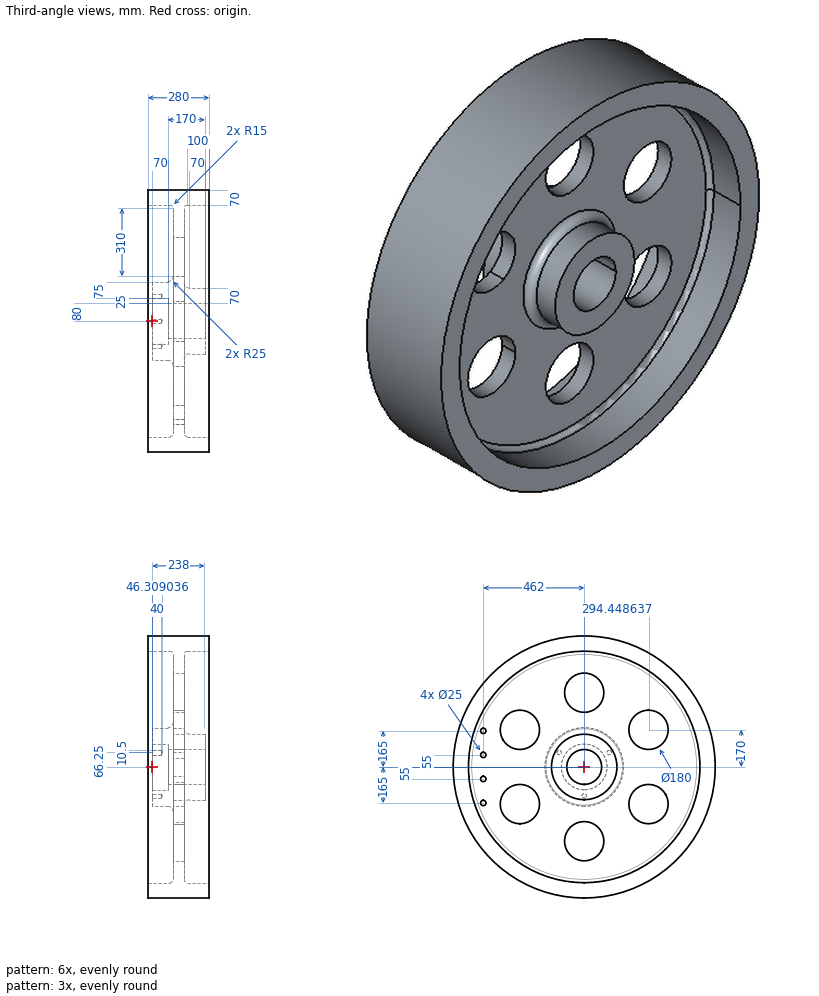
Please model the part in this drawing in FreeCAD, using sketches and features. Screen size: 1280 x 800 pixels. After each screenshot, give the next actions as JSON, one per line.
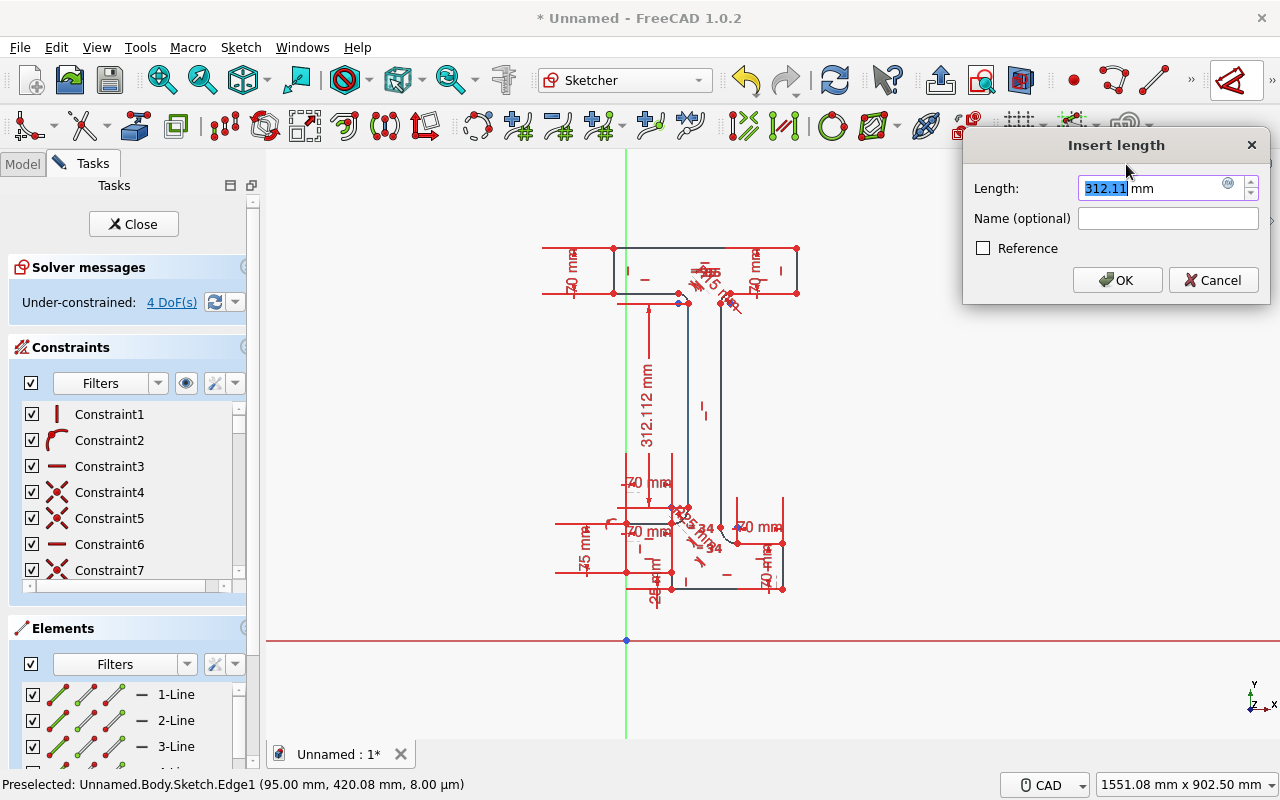
{"action": "type", "text": "310"}
{"action": "key", "text": "Return"}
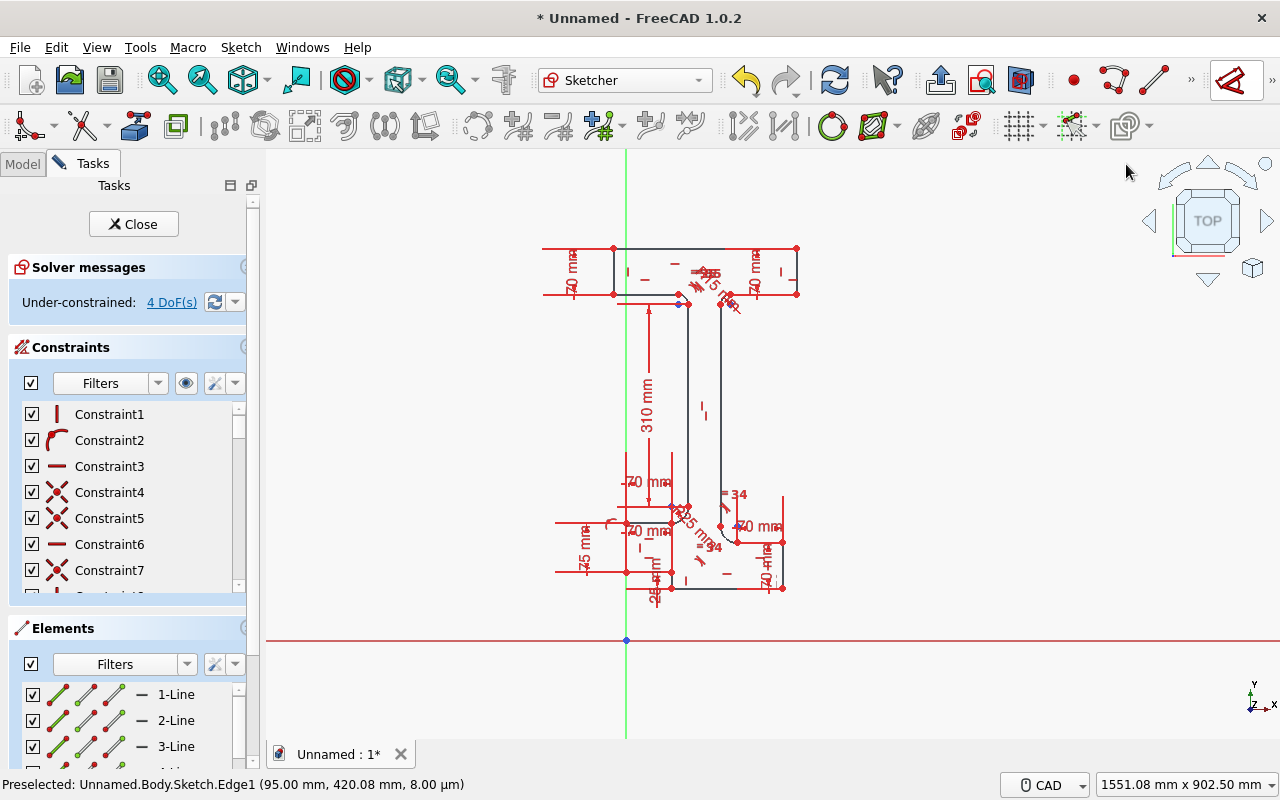
{"action": "left_click", "coordinate": [705, 589]}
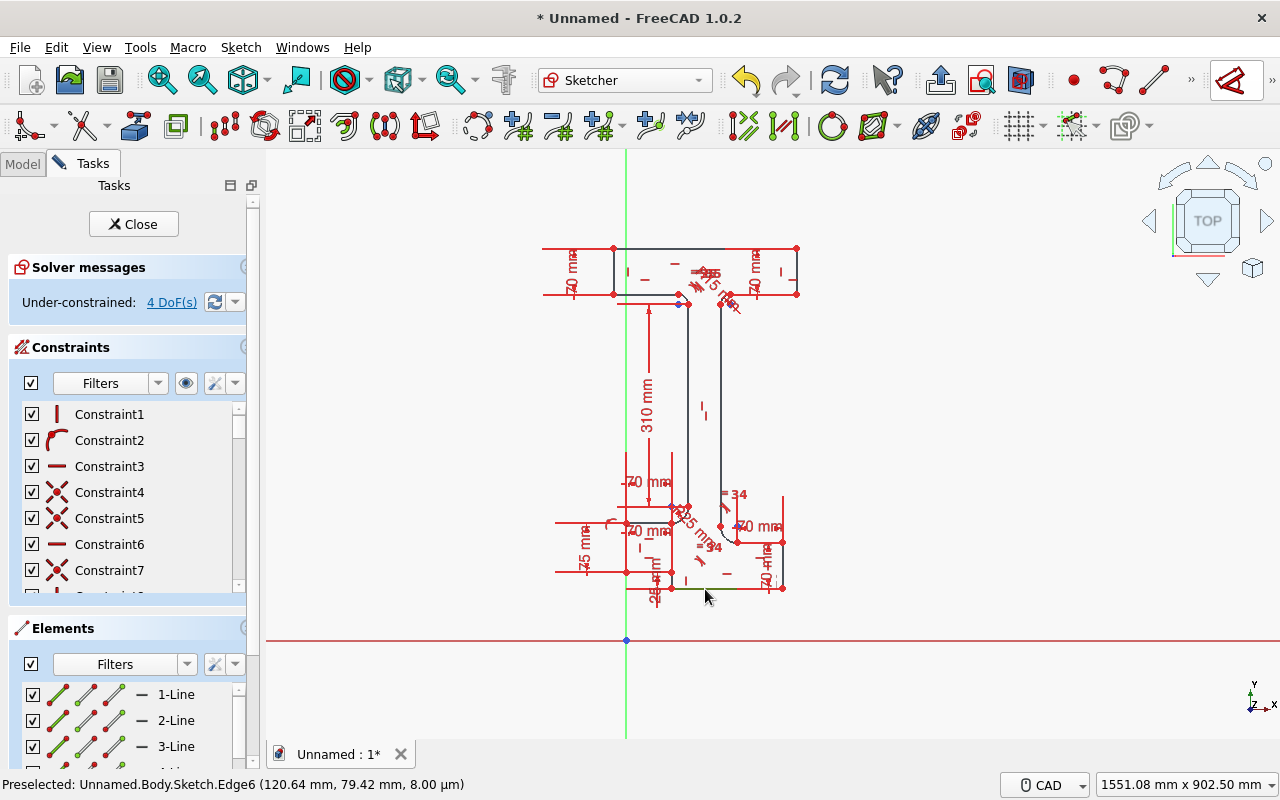
{"action": "left_click", "coordinate": [1258, 80]}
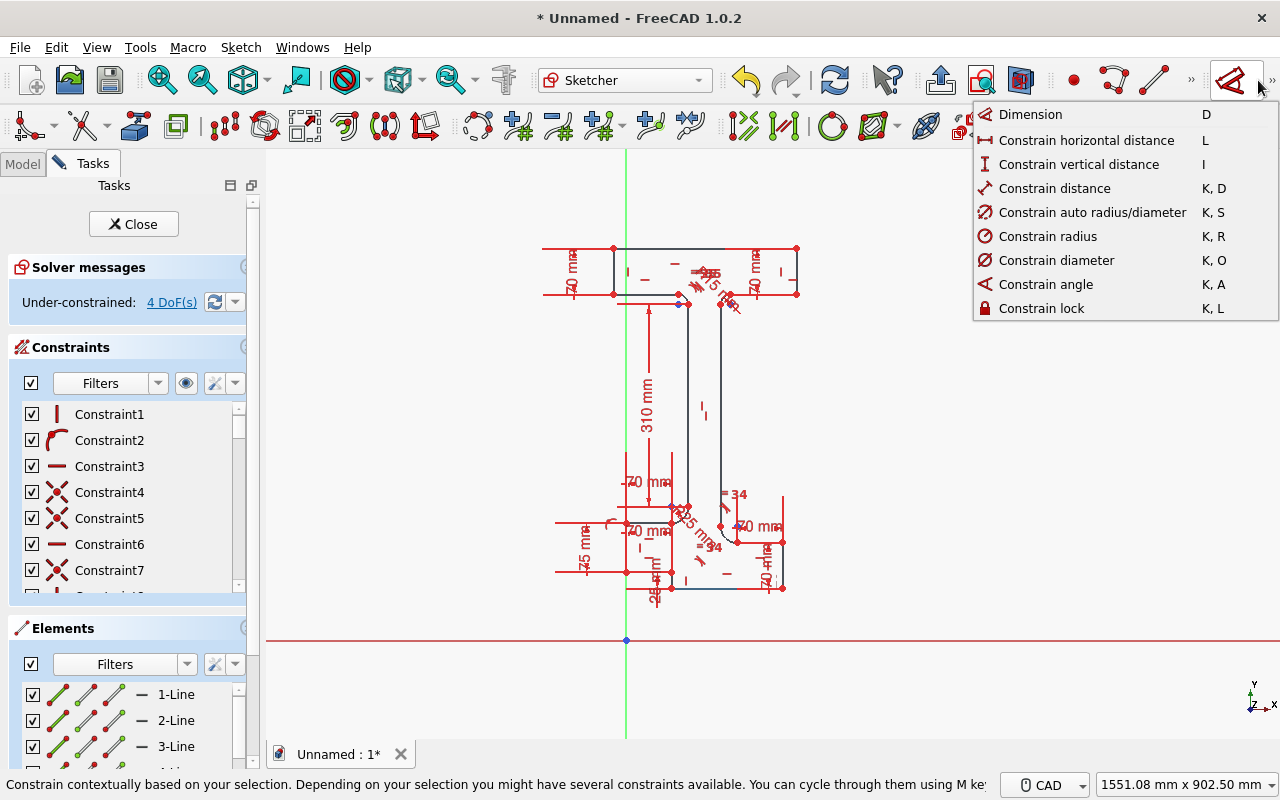
{"action": "left_click", "coordinate": [1126, 140]}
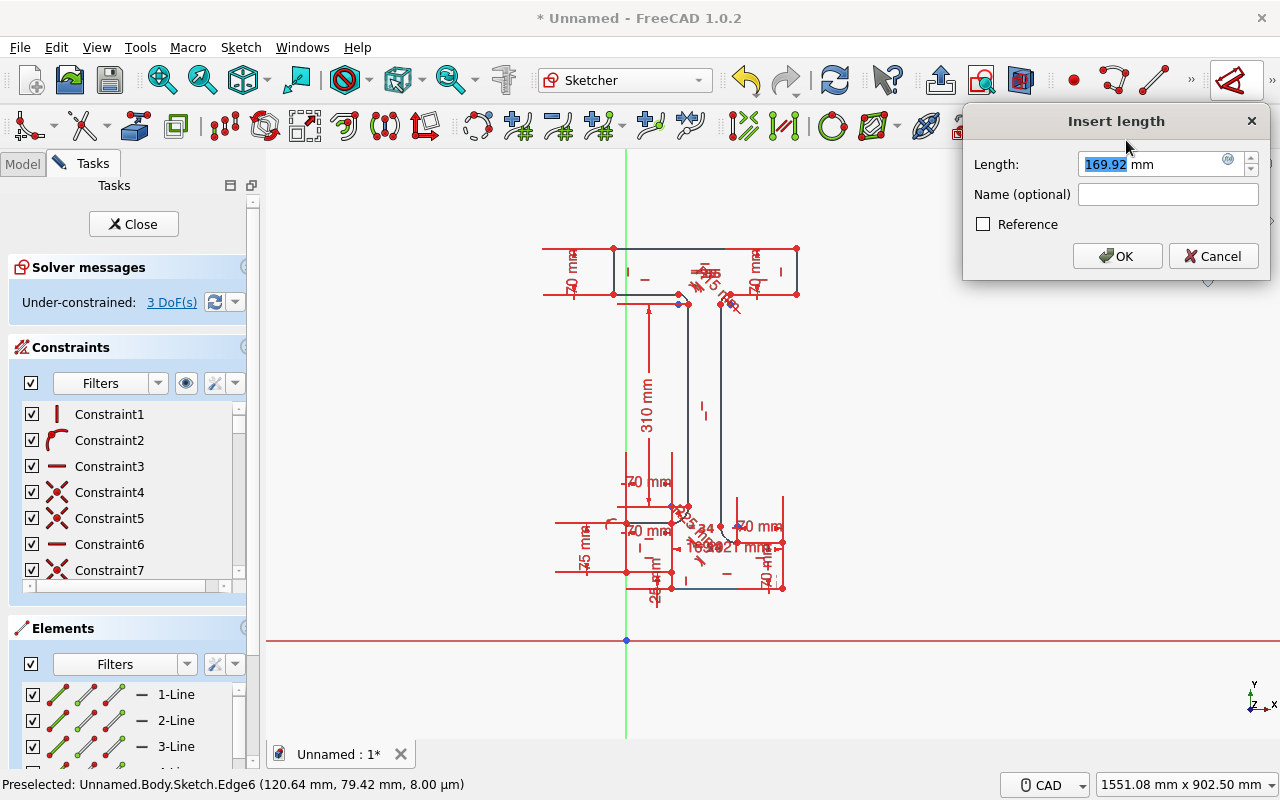
{"action": "type", "text": "170"}
{"action": "key", "text": "Return"}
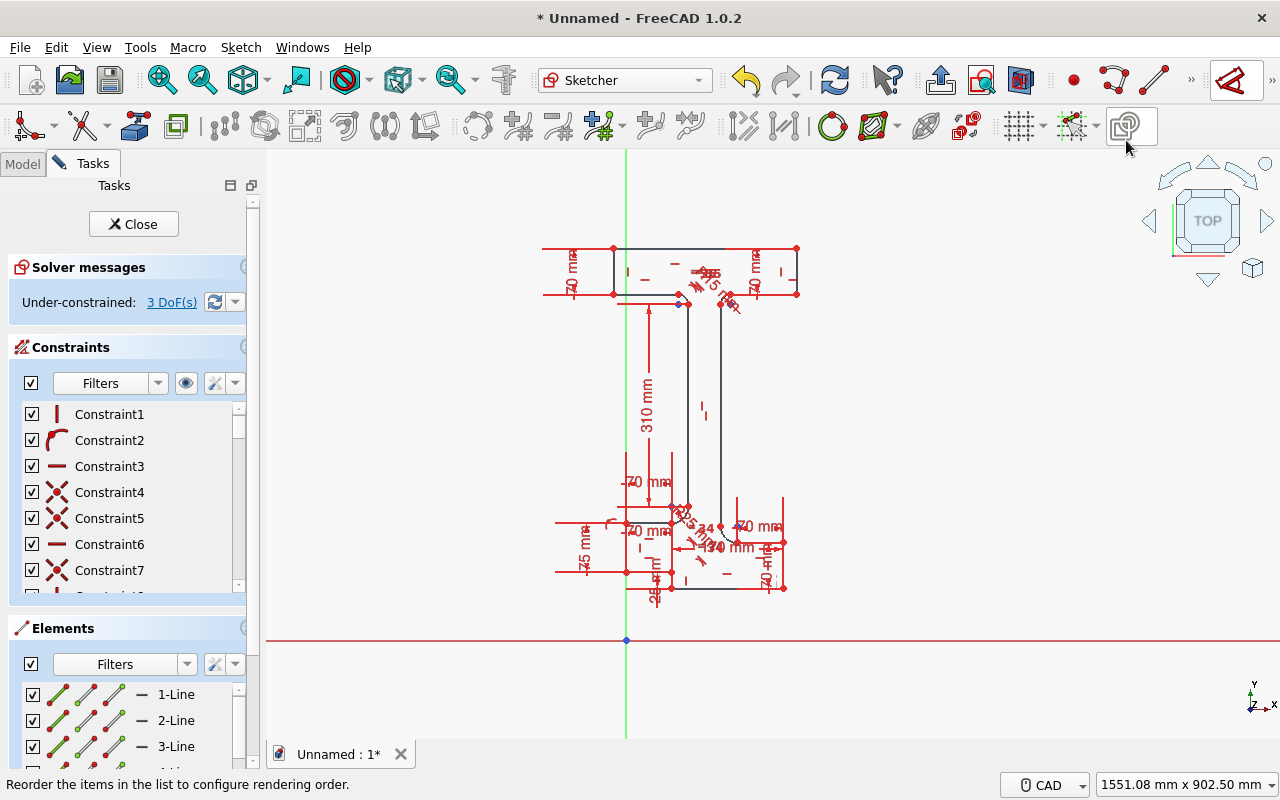
{"action": "left_click", "coordinate": [750, 295]}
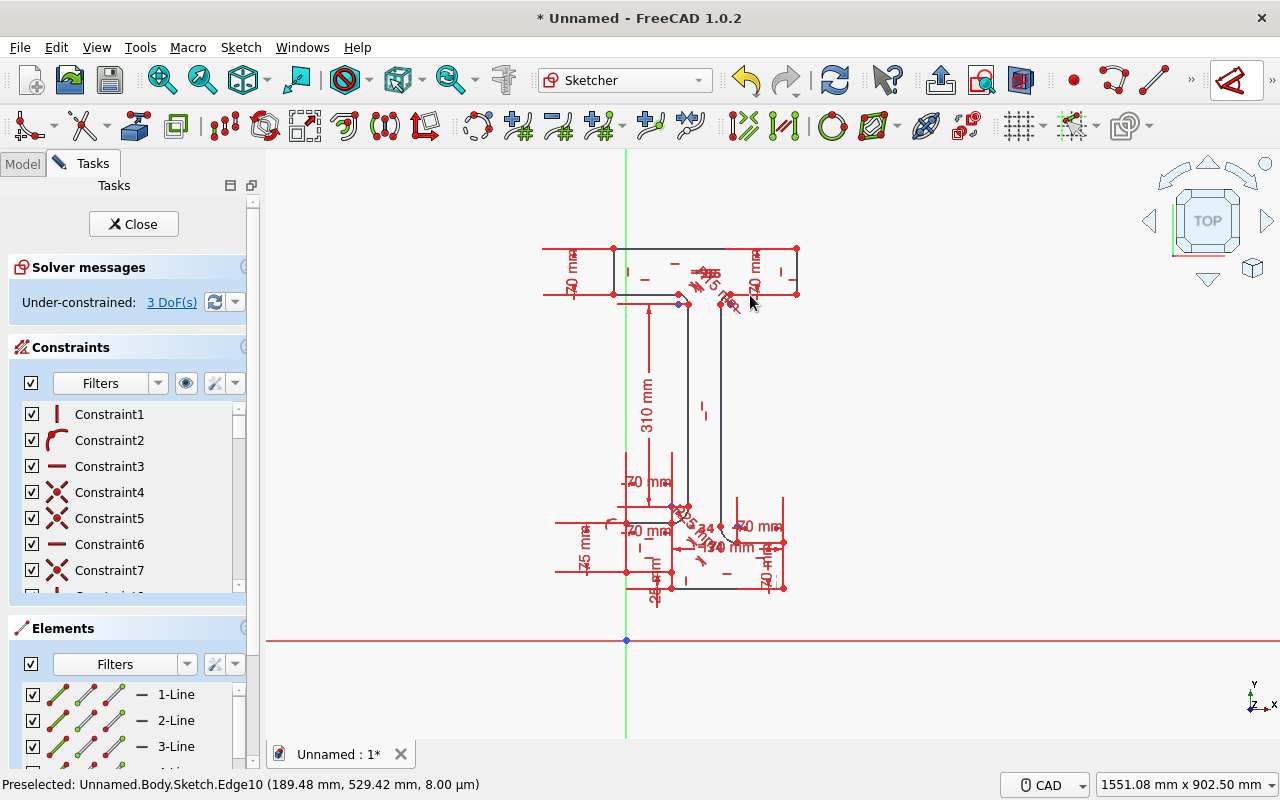
{"action": "left_click", "coordinate": [1258, 80]}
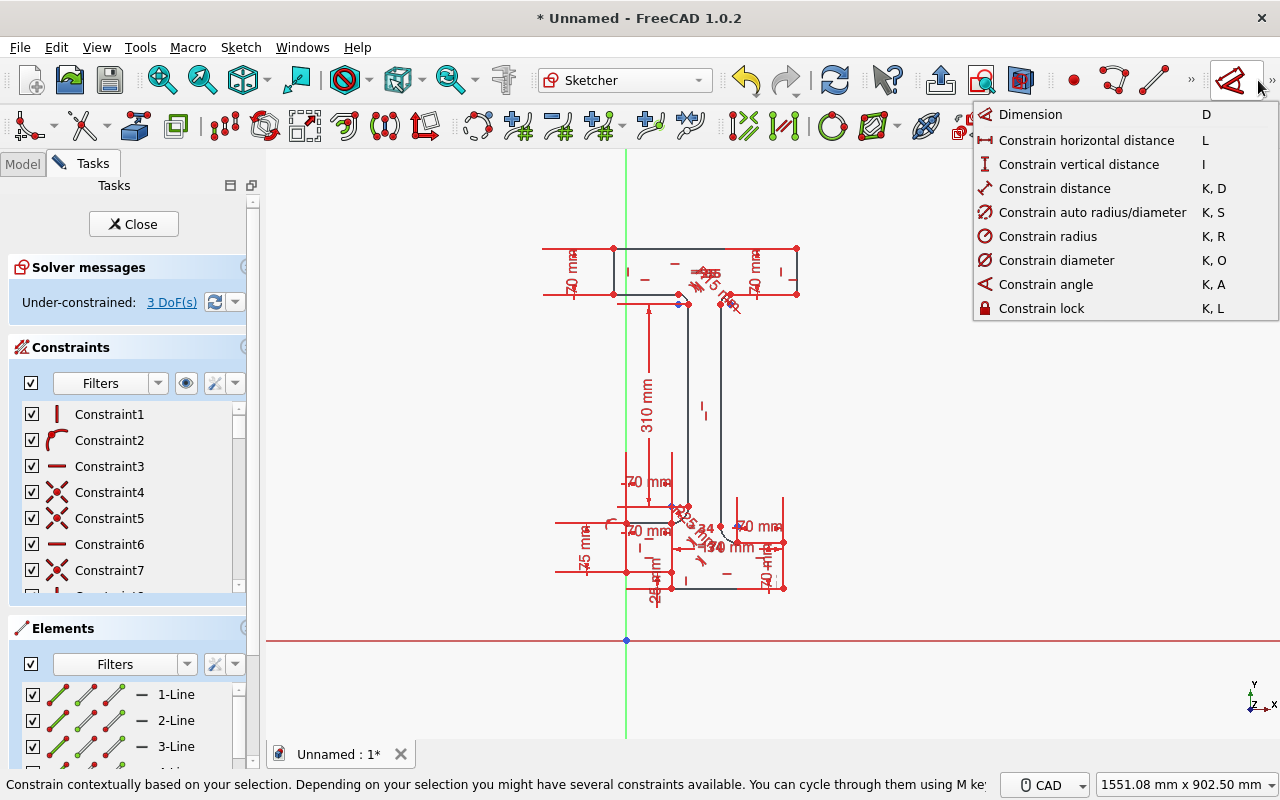
{"action": "left_click", "coordinate": [1126, 140]}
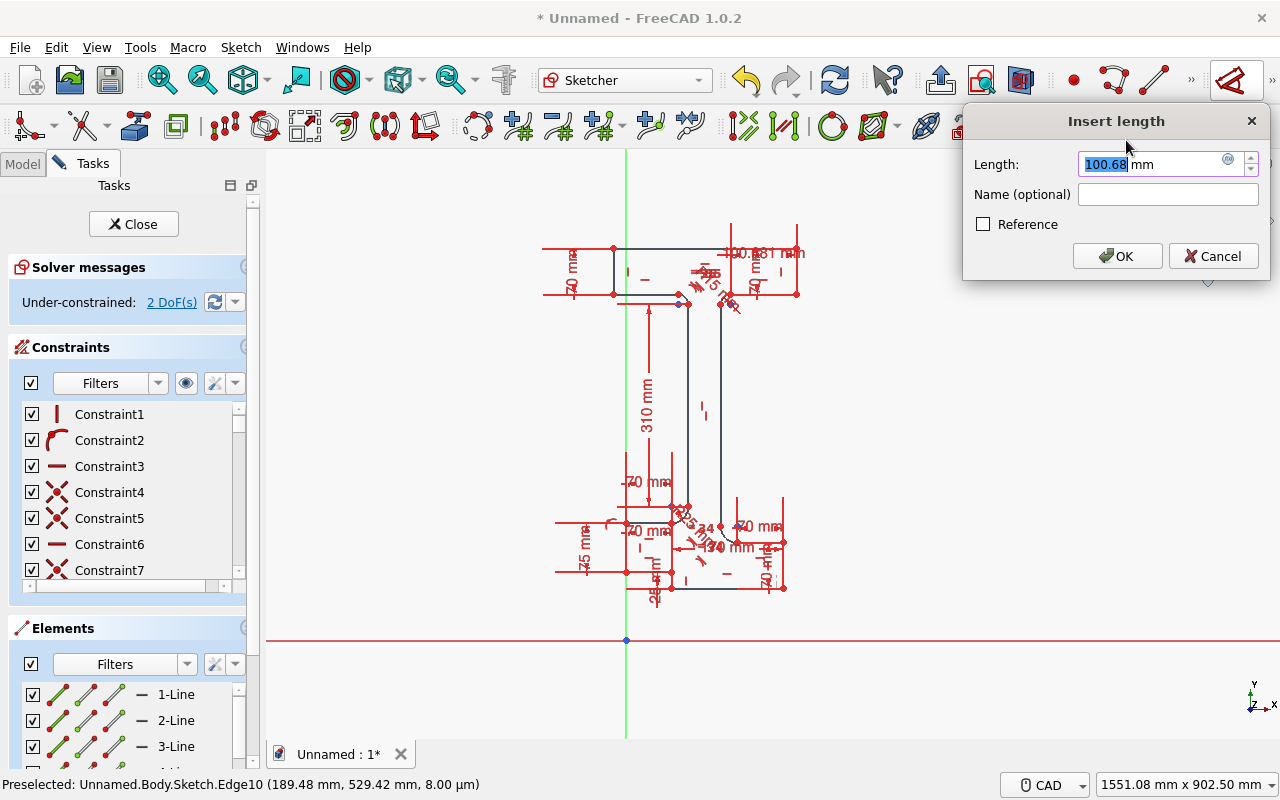
{"action": "type", "text": "100"}
{"action": "key", "text": "Return"}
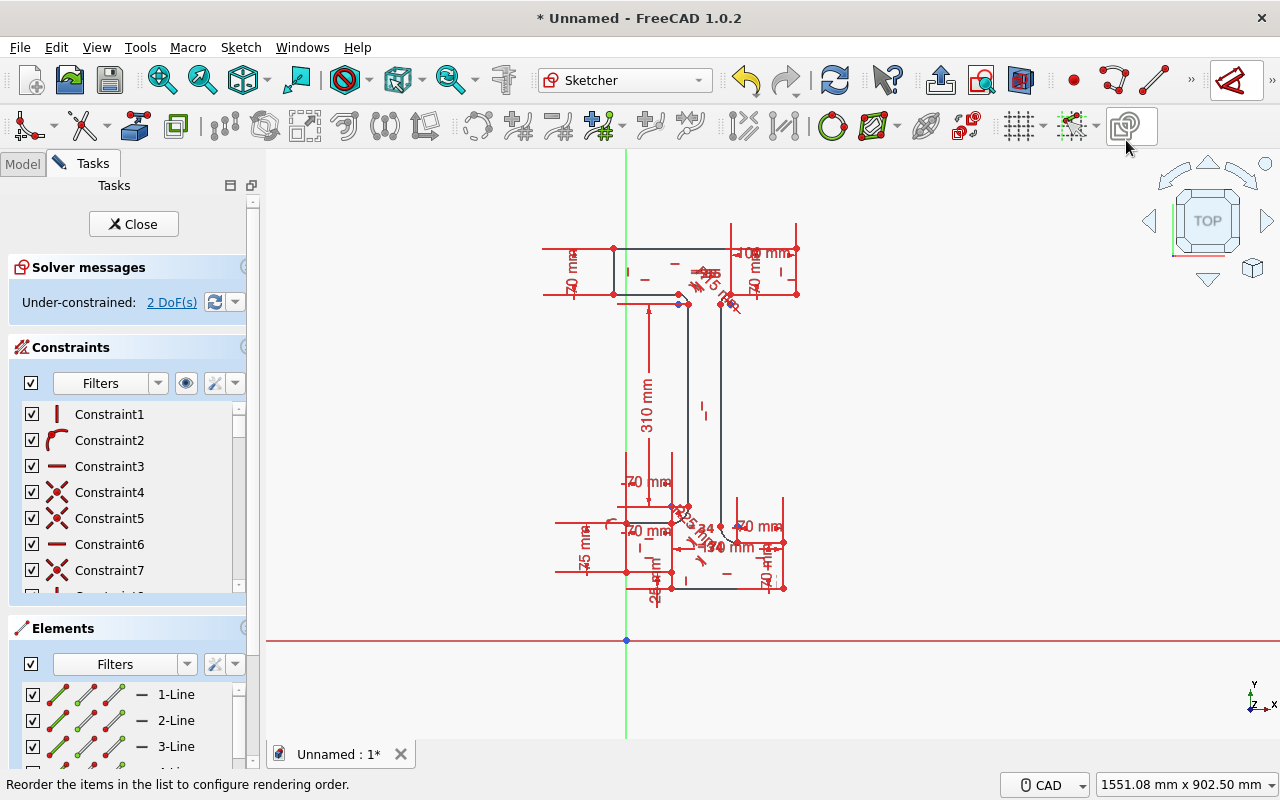
{"action": "left_click", "coordinate": [668, 249]}